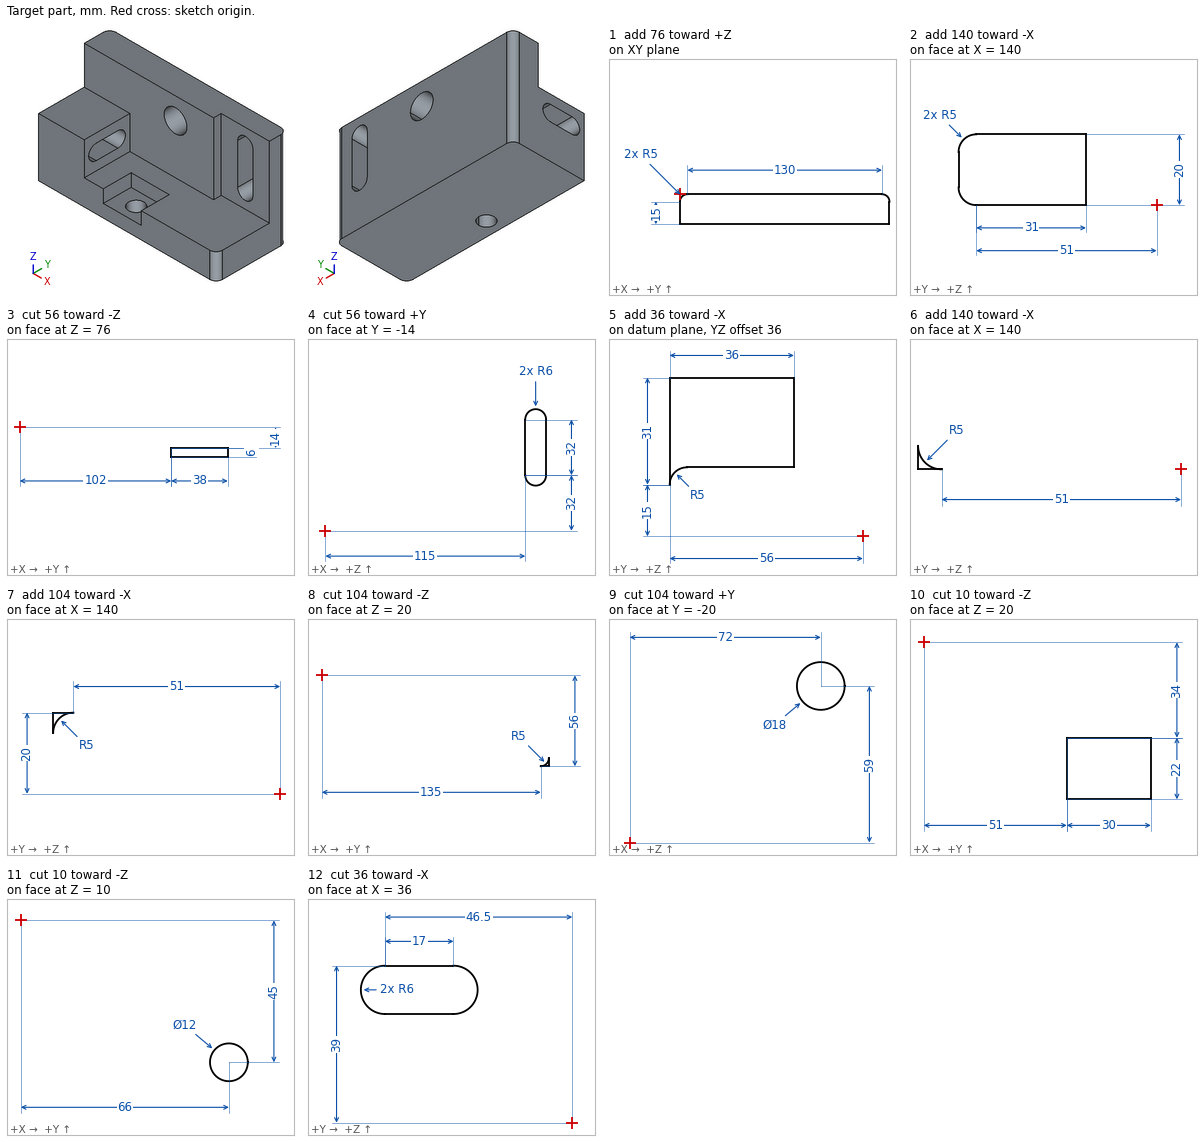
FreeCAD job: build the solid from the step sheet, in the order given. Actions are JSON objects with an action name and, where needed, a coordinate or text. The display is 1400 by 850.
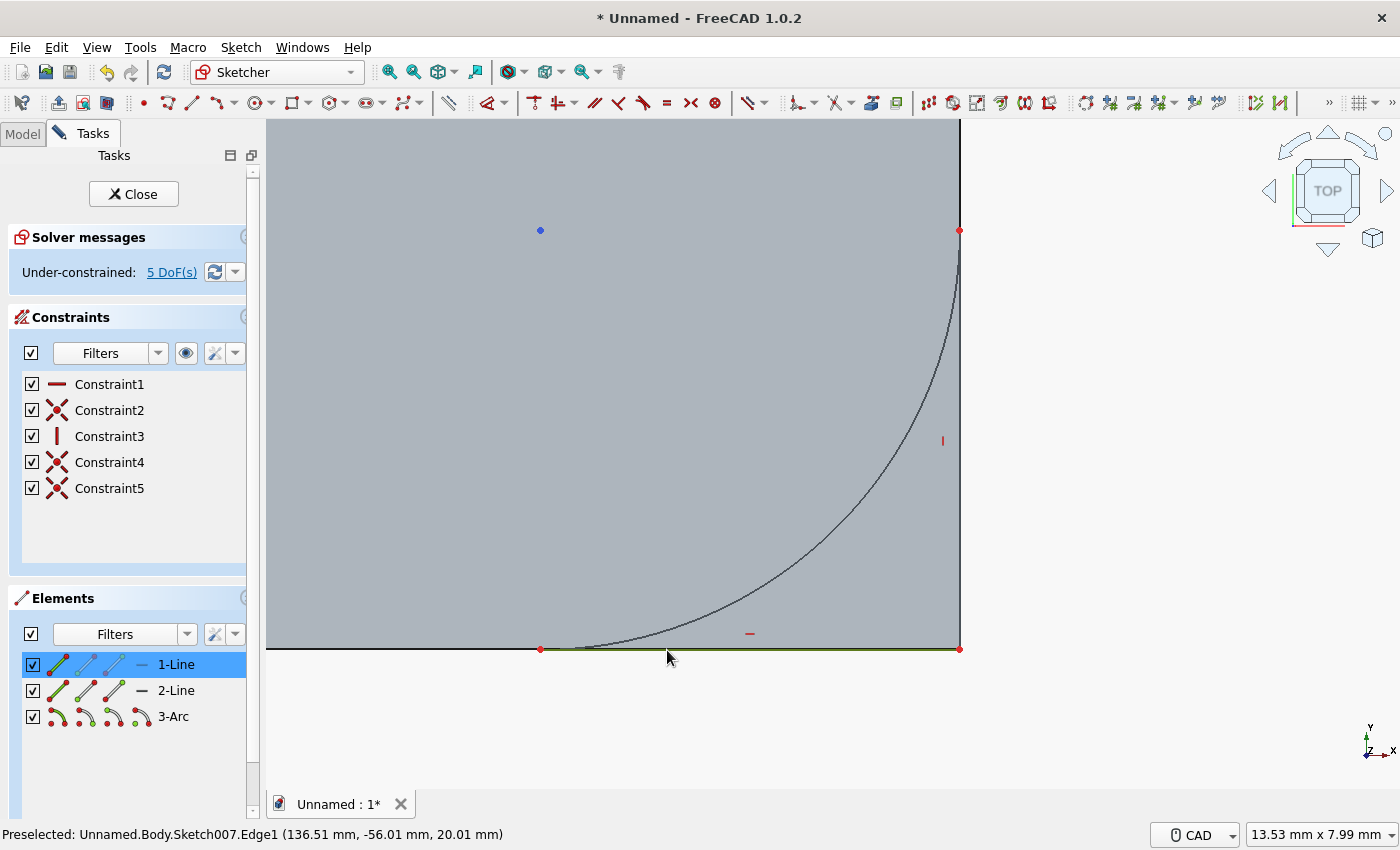
{"action": "left_click", "coordinate": [731, 604]}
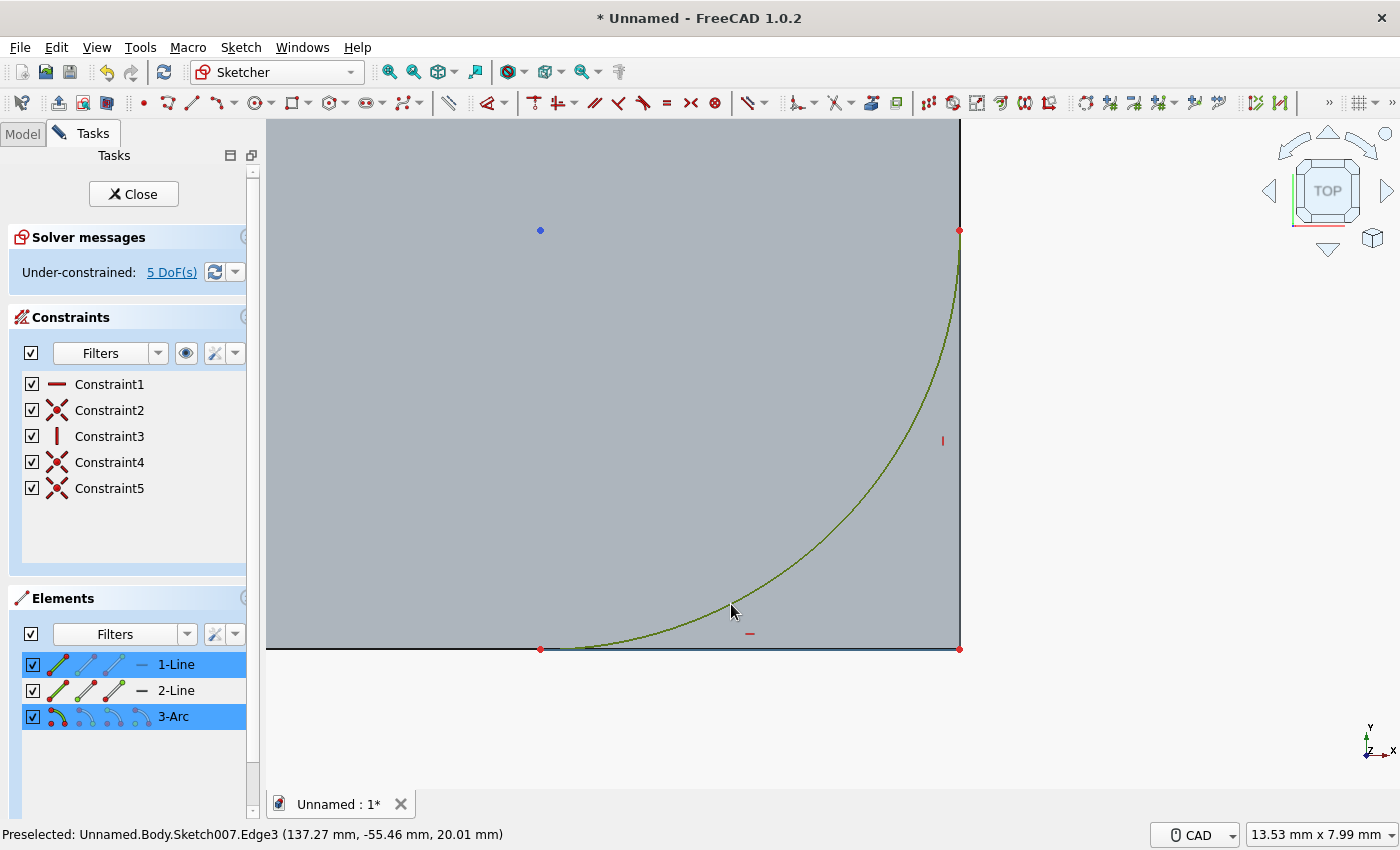
{"action": "key", "text": "t"}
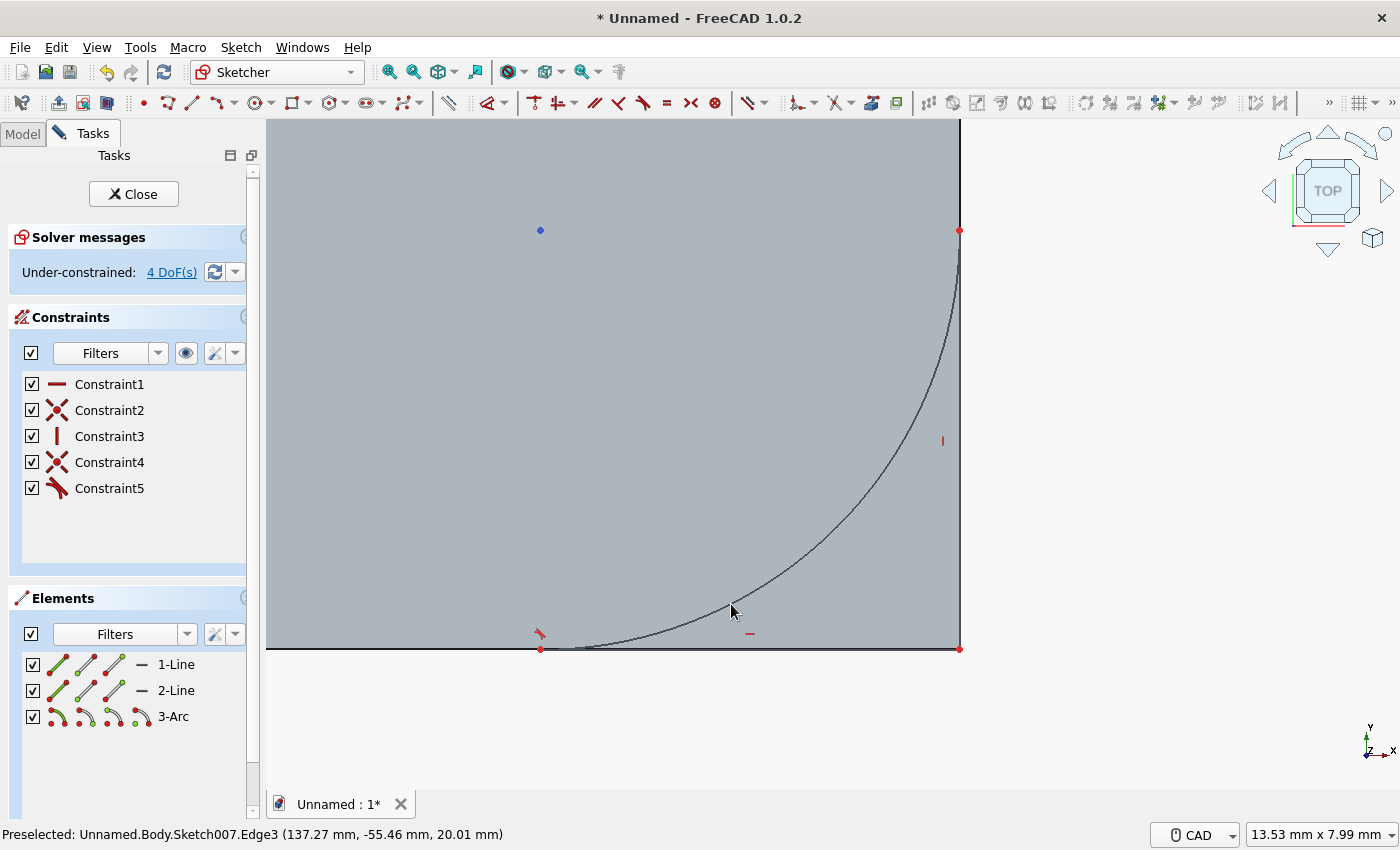
{"action": "left_click", "coordinate": [960, 524]}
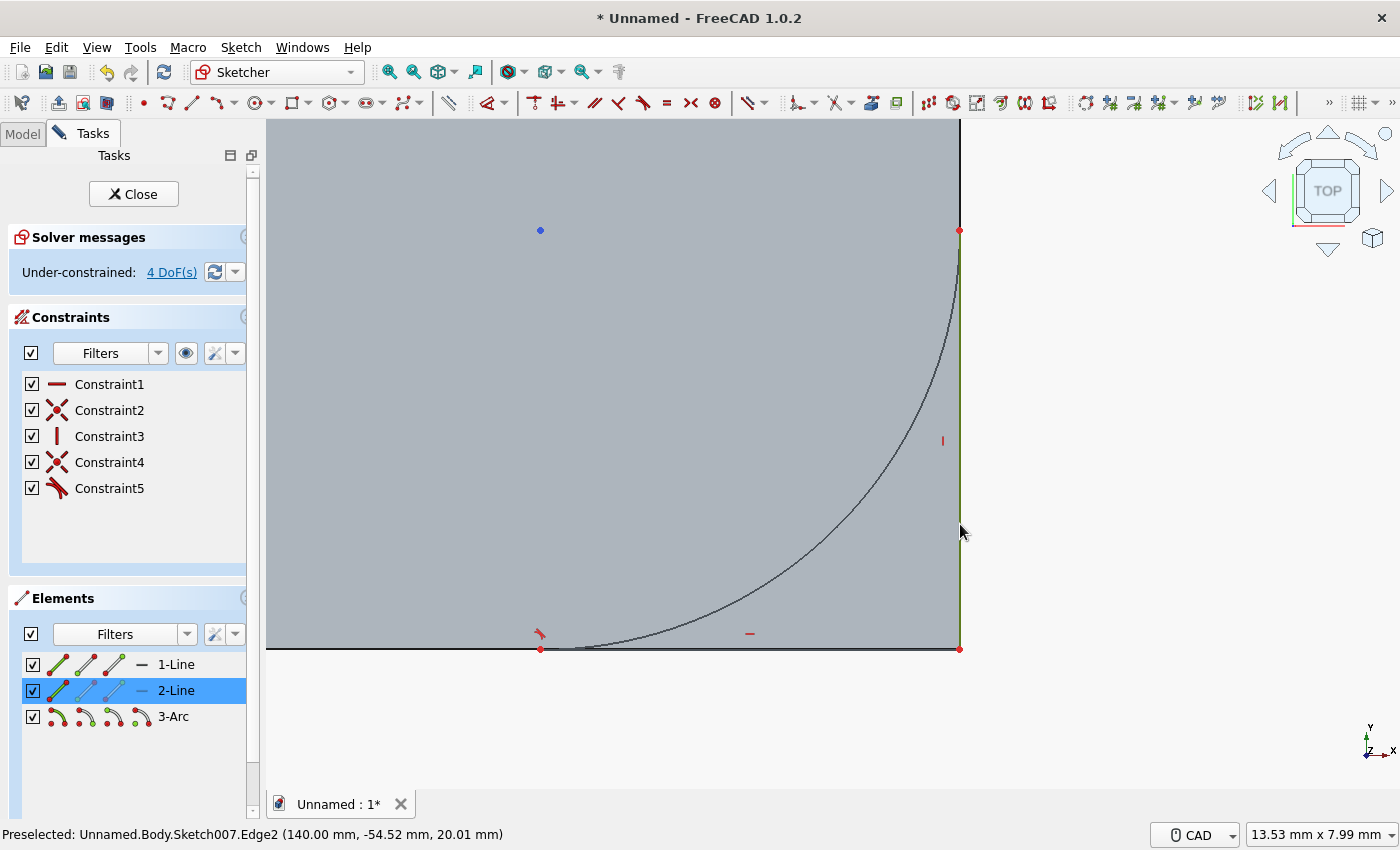
{"action": "left_click", "coordinate": [730, 604]}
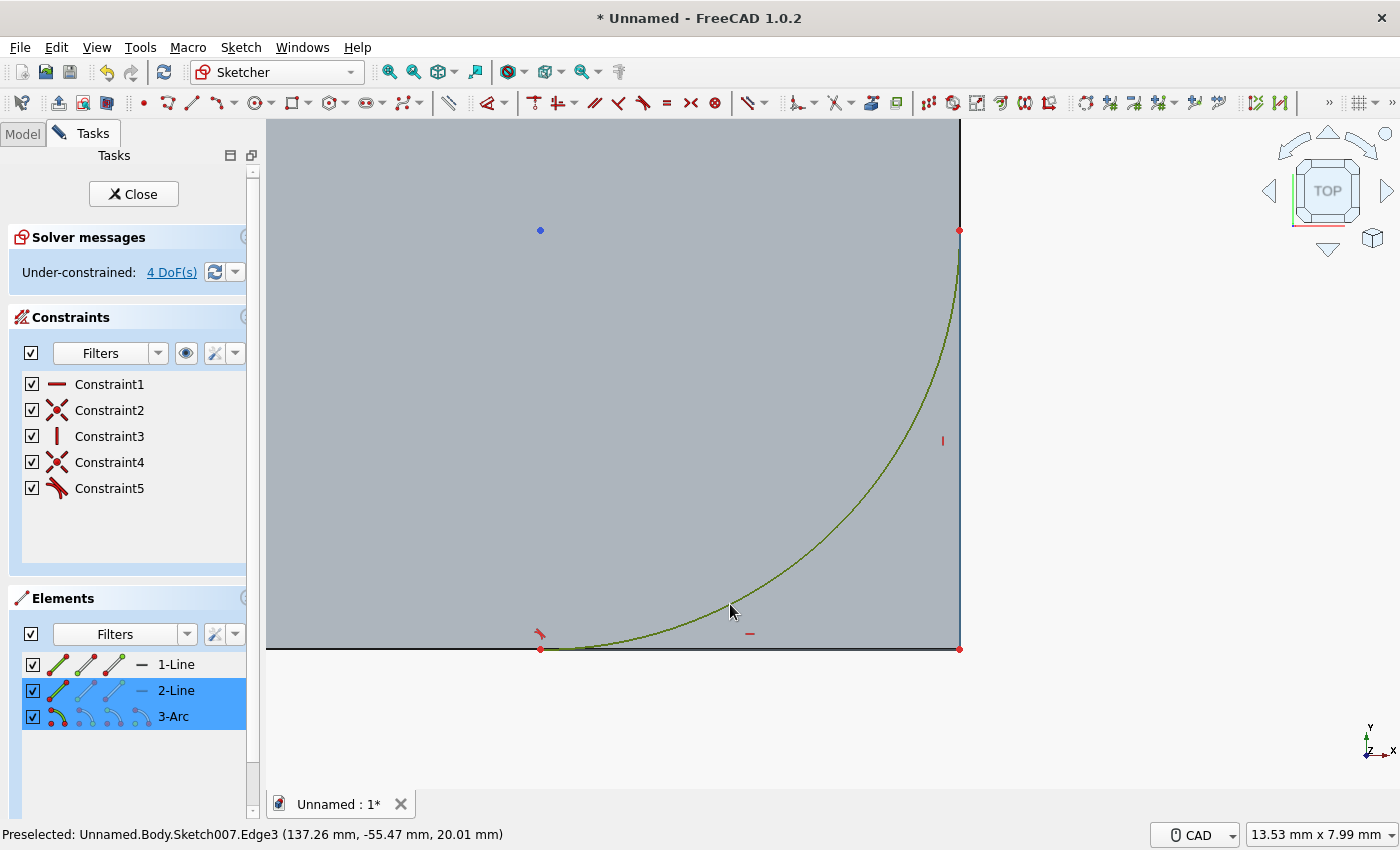
{"action": "left_click", "coordinate": [644, 104]}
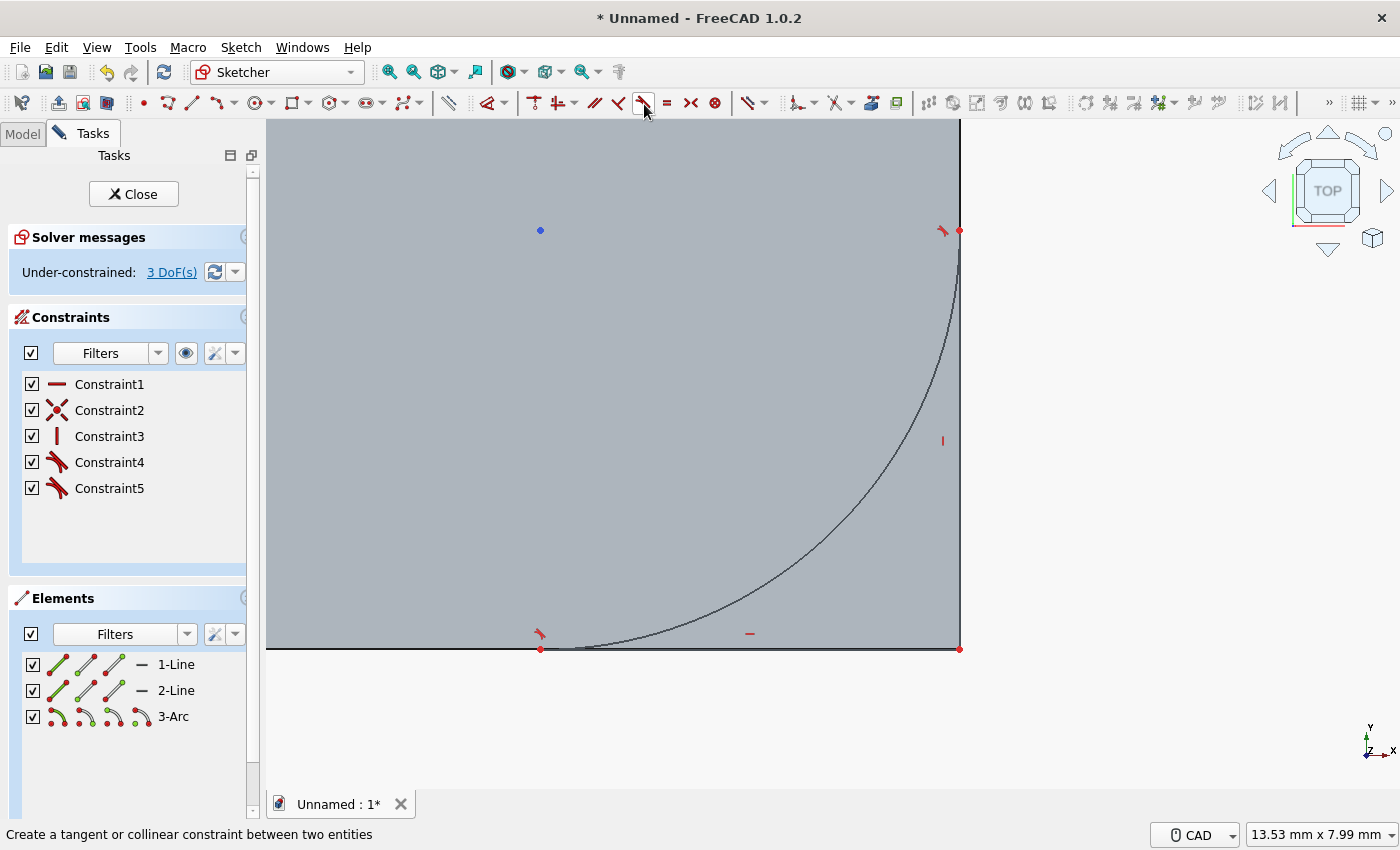
{"action": "left_click", "coordinate": [488, 104]}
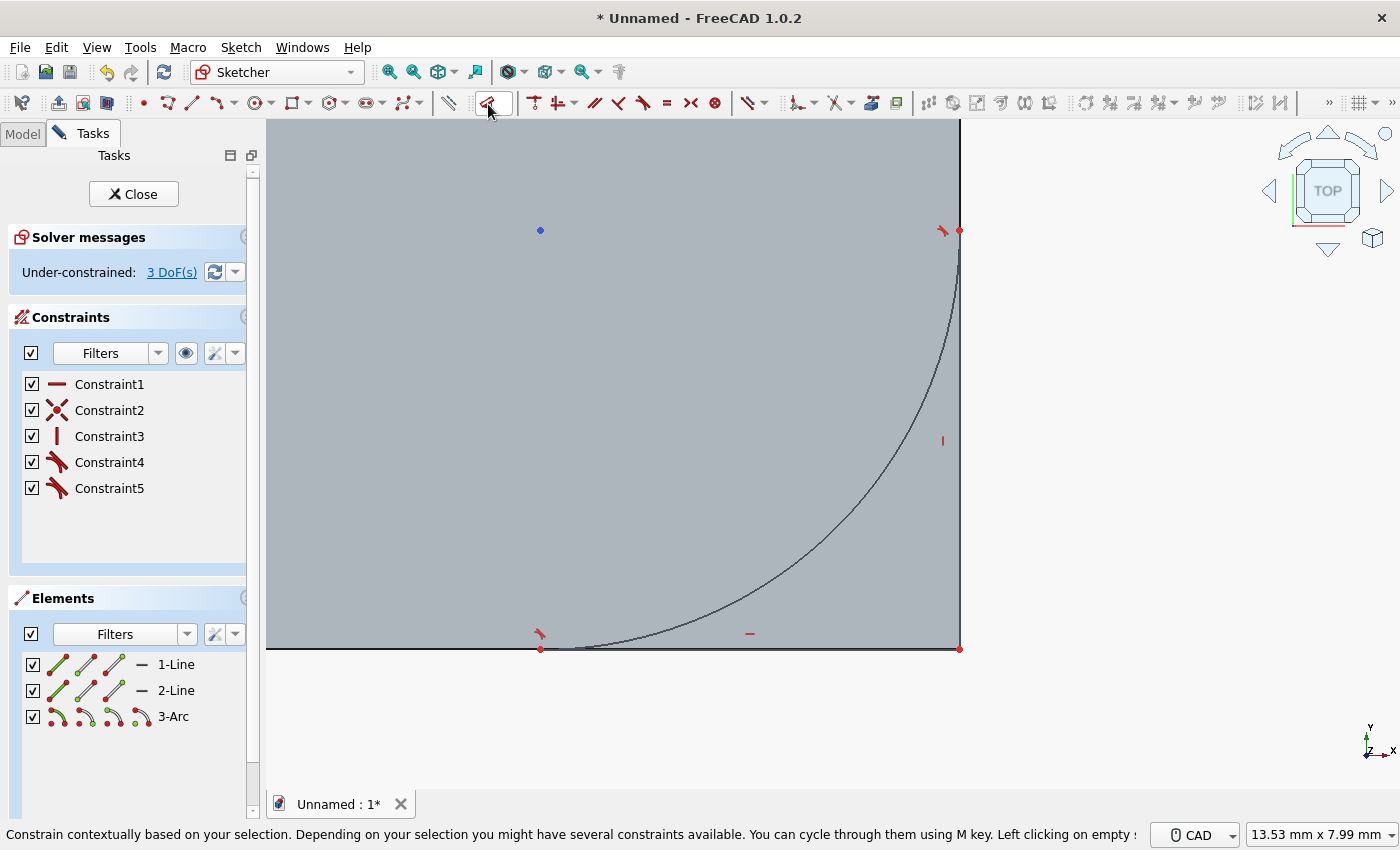
{"action": "left_click", "coordinate": [731, 604]}
{"action": "left_click", "coordinate": [746, 632]}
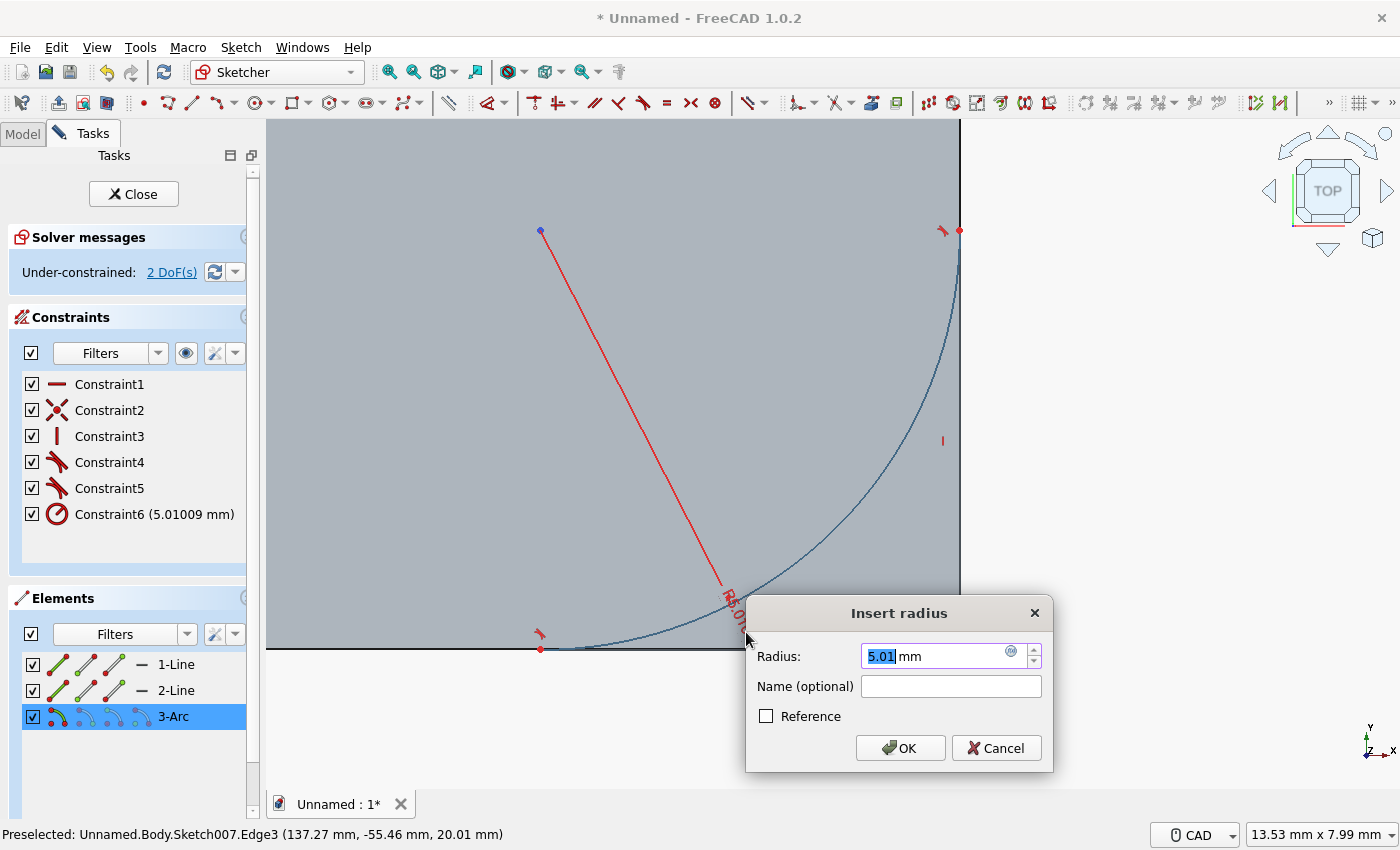
{"action": "type", "text": "5"}
{"action": "key", "text": "Return"}